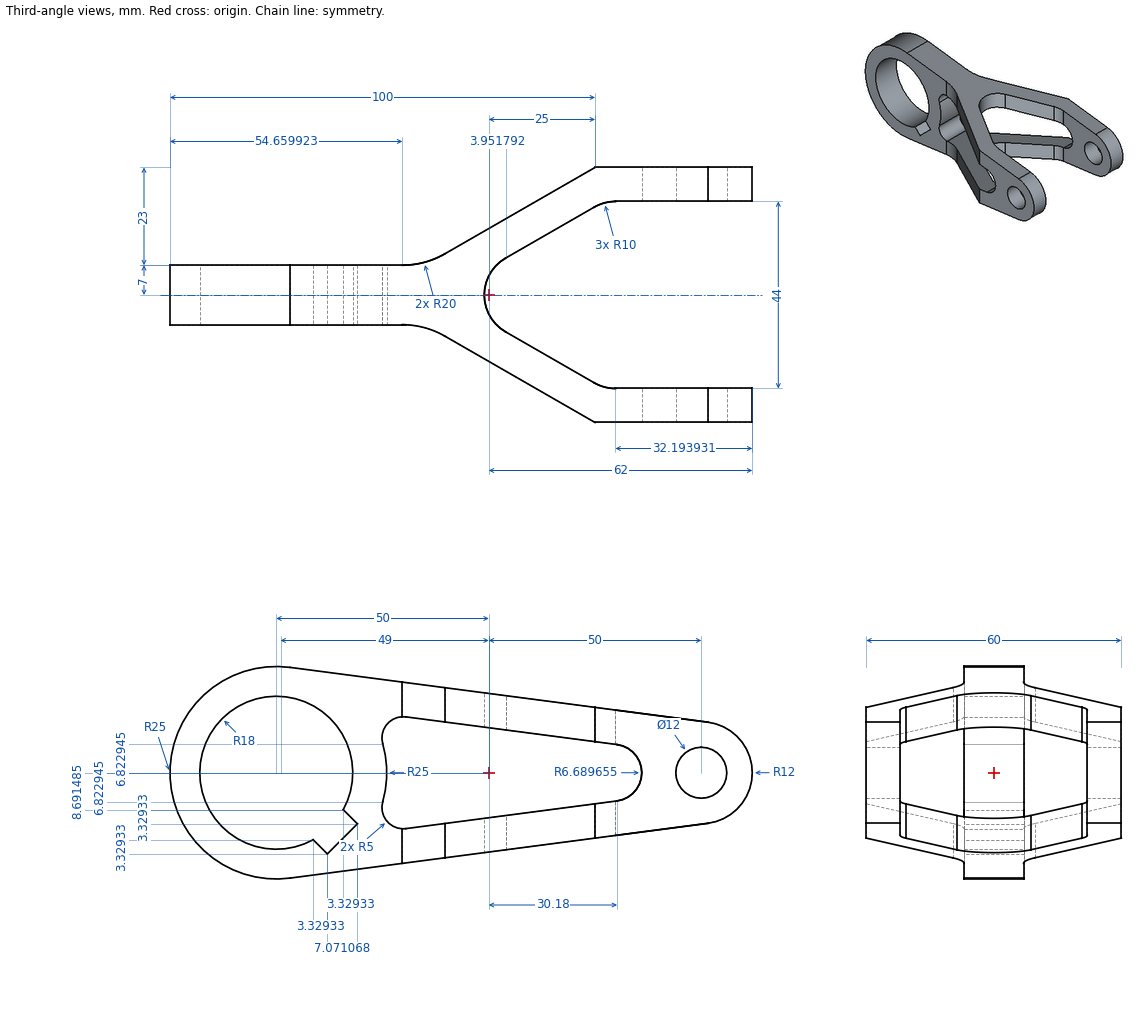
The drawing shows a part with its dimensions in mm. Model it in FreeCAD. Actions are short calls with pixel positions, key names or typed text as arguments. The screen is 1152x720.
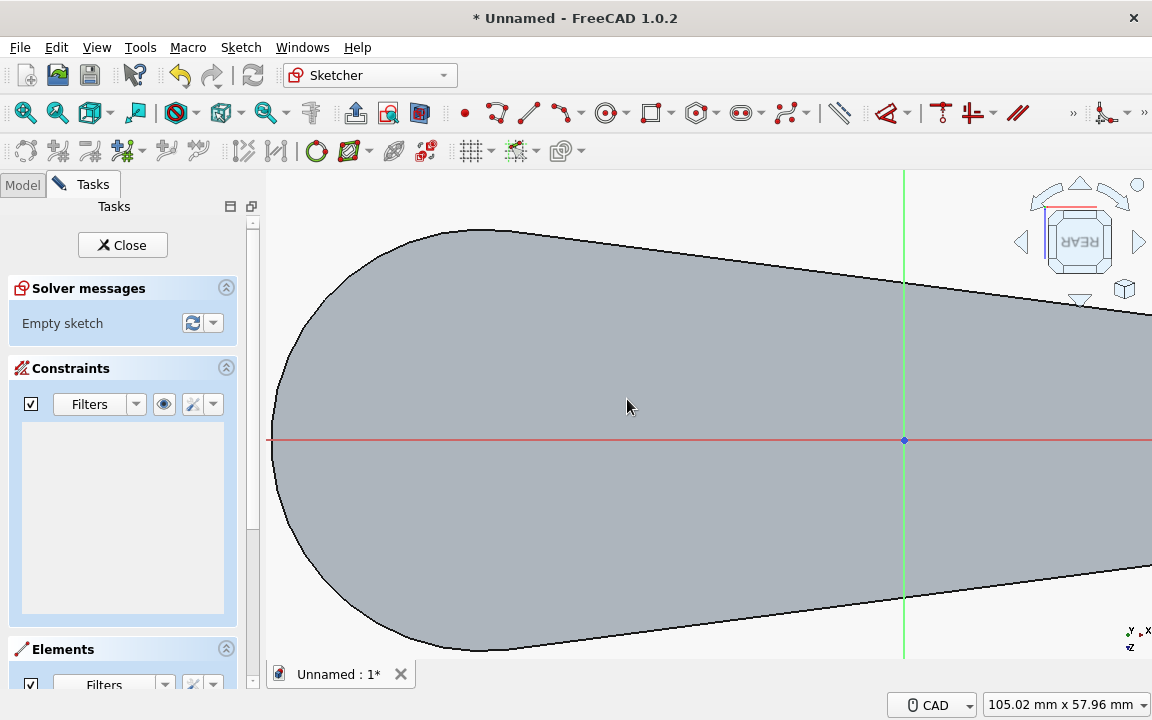
click(498, 114)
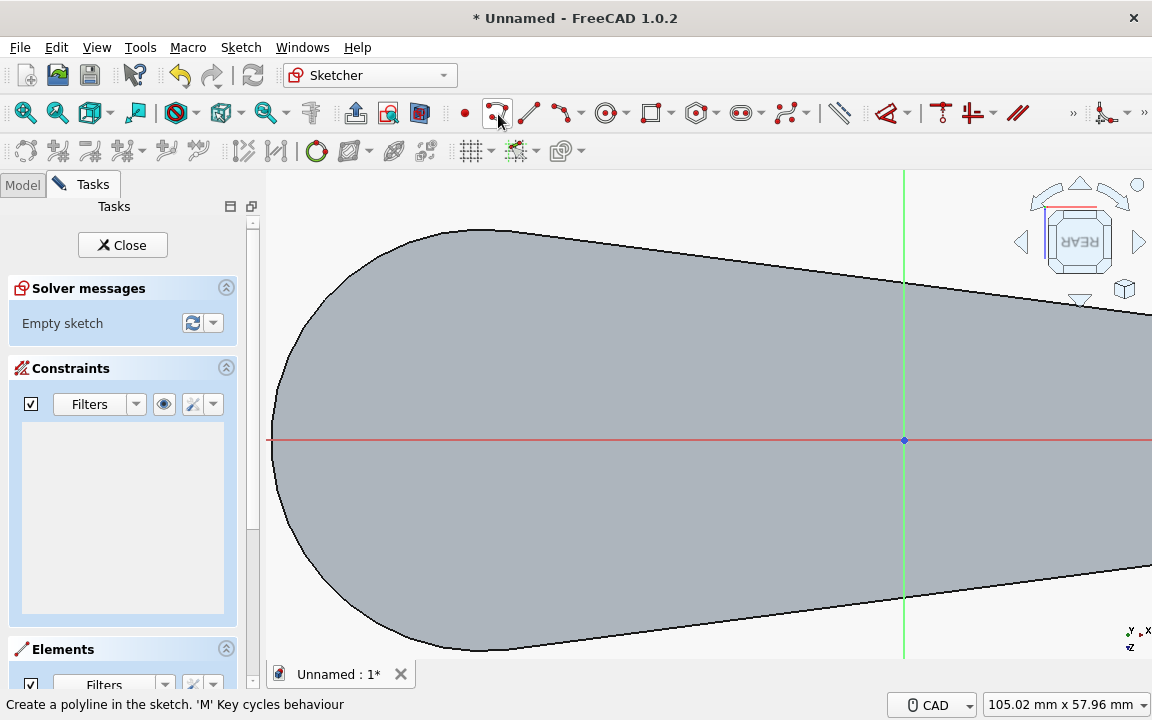
click(615, 367)
click(643, 339)
click(584, 279)
click(555, 307)
right_click(555, 307)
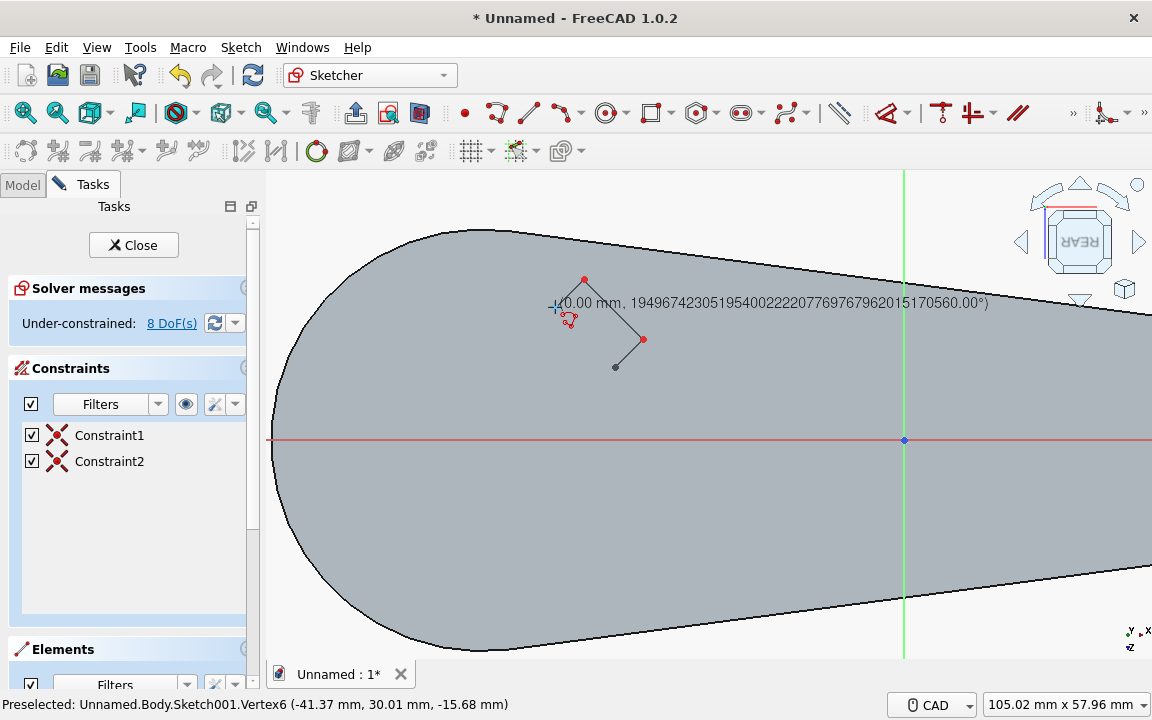
click(562, 114)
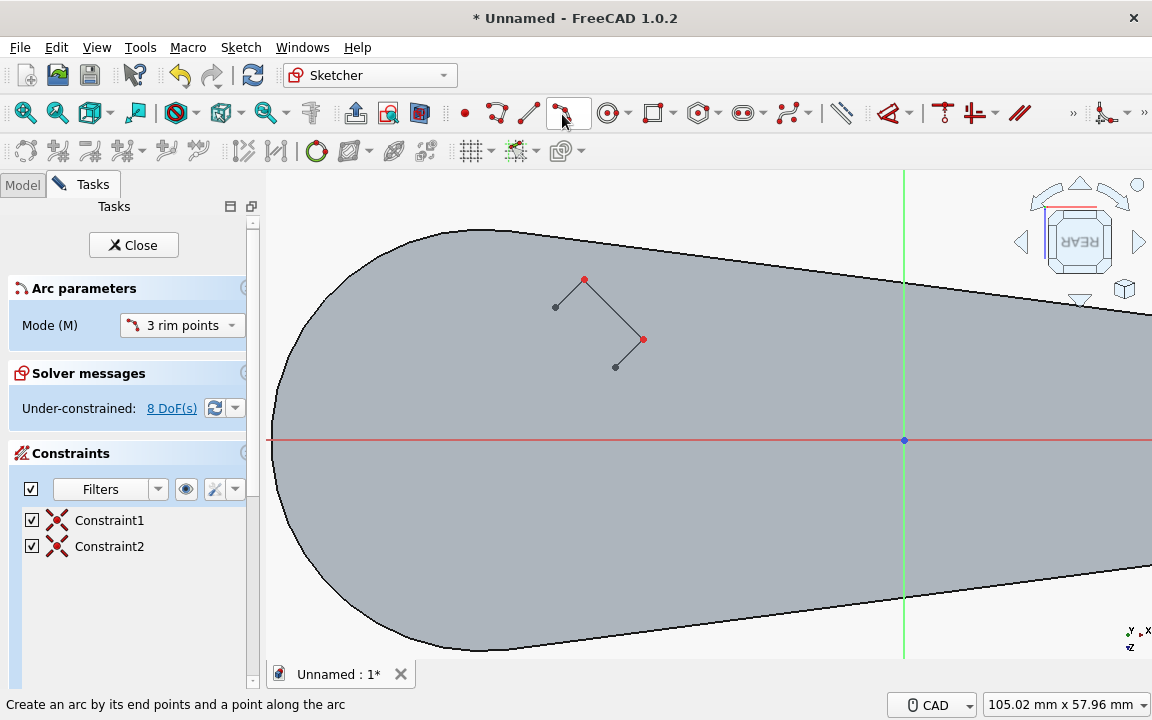
click(555, 308)
click(615, 368)
click(375, 548)
key(Escape)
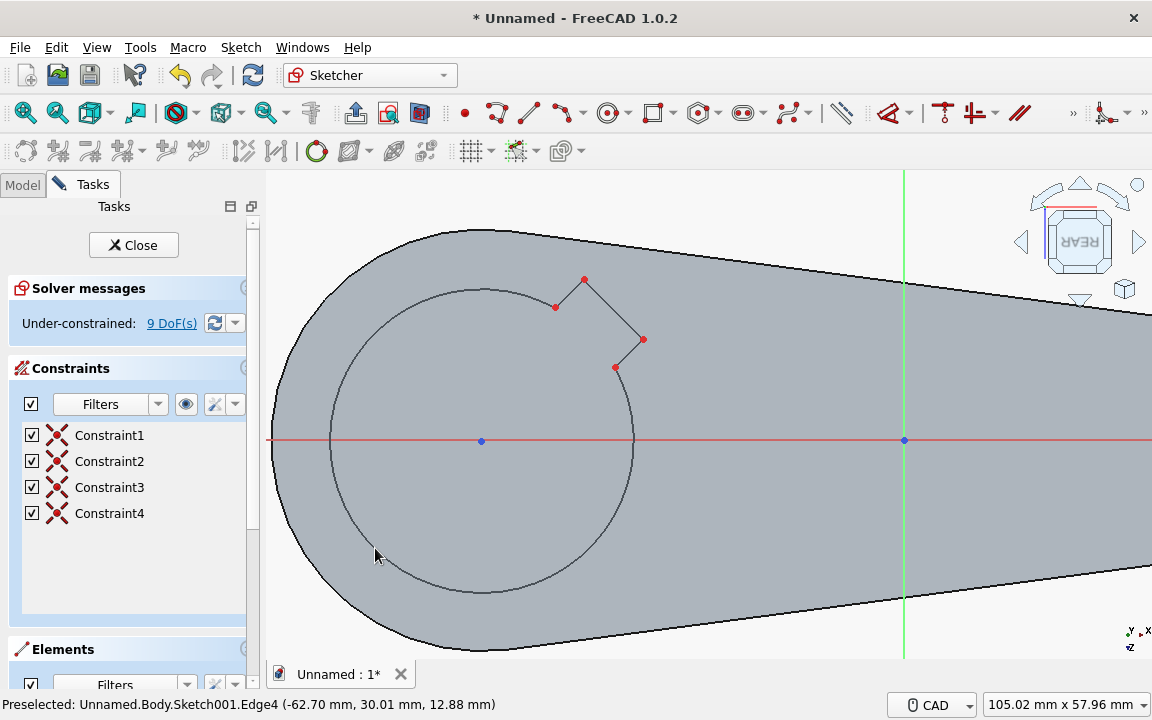
click(482, 441)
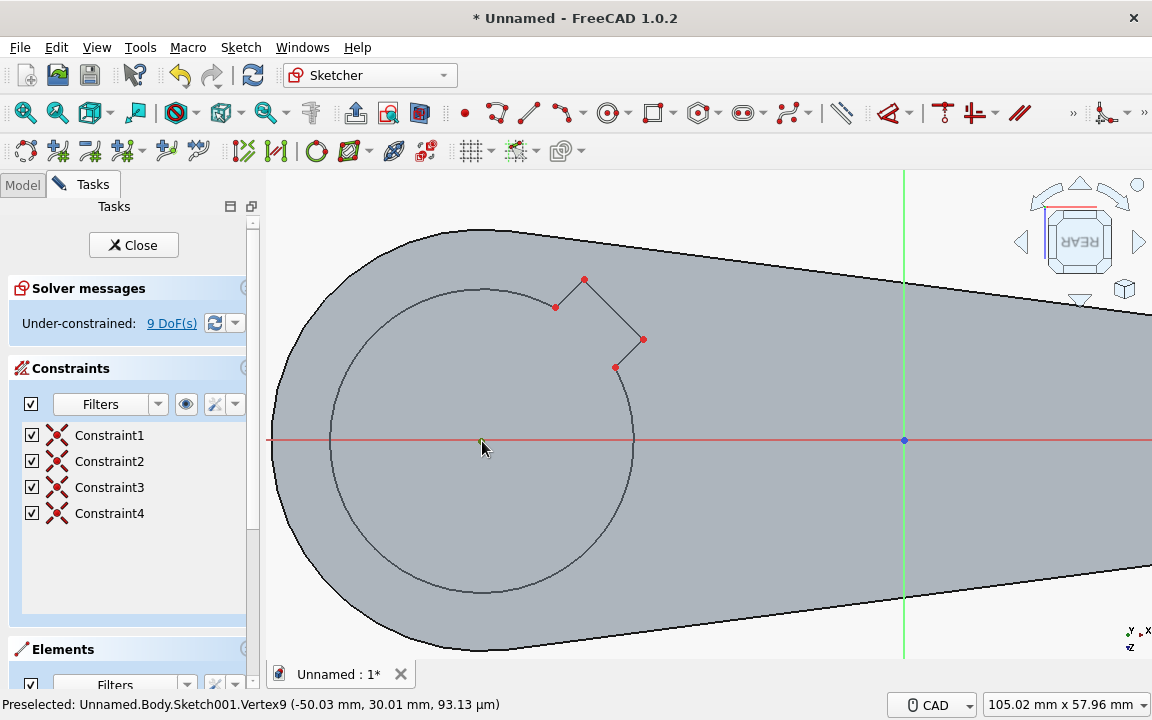
click(393, 440)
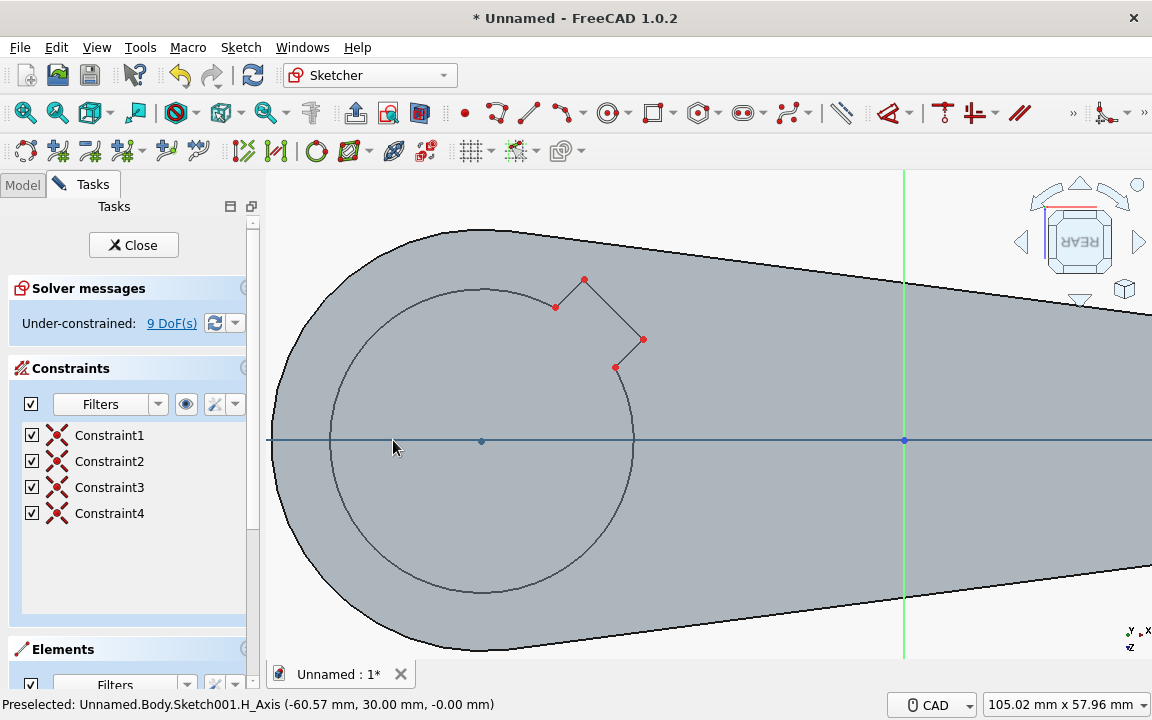
click(944, 114)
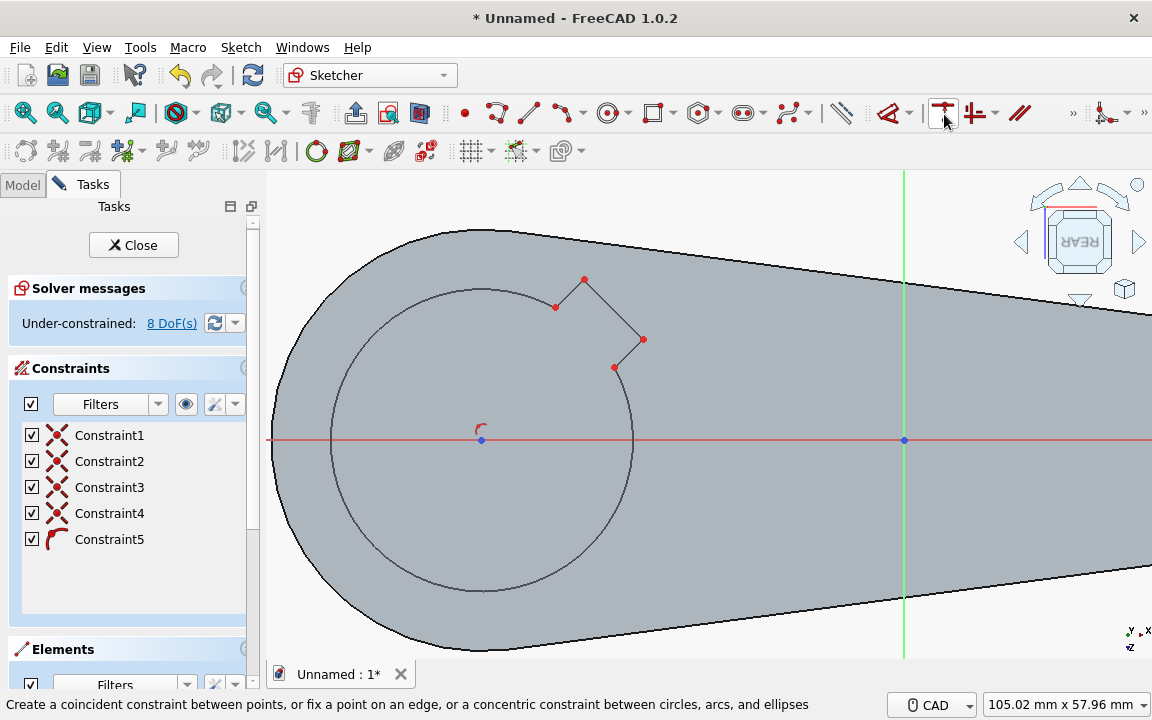
click(888, 114)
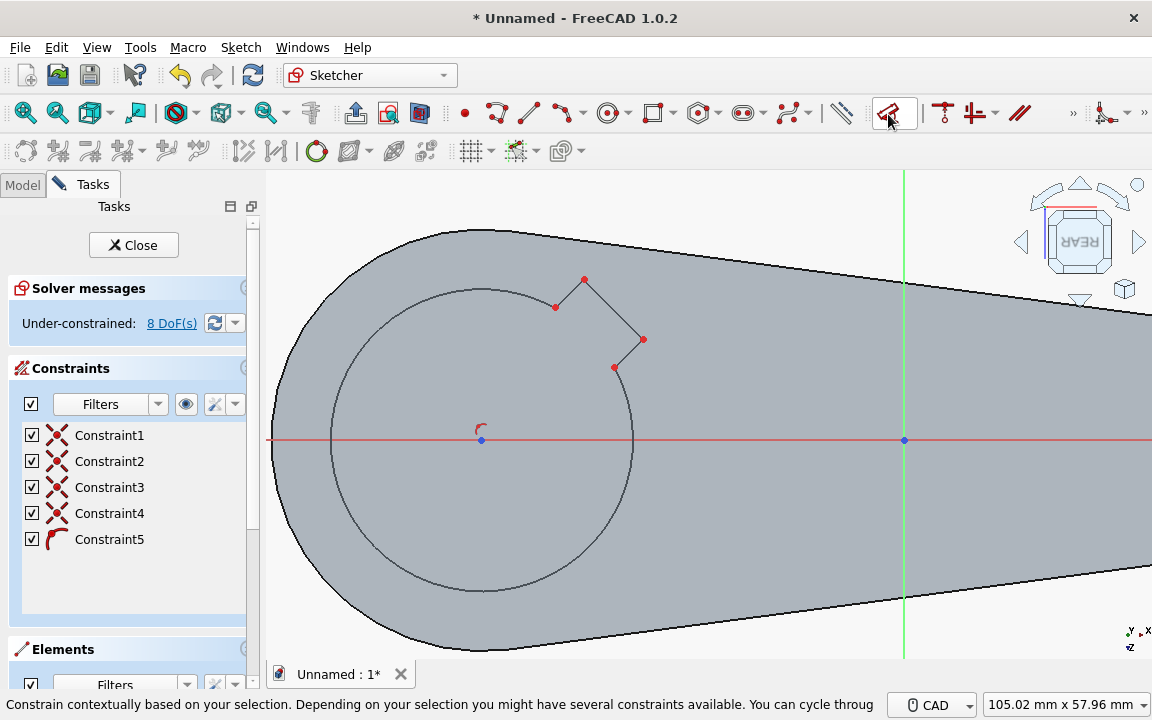
click(340, 387)
click(310, 376)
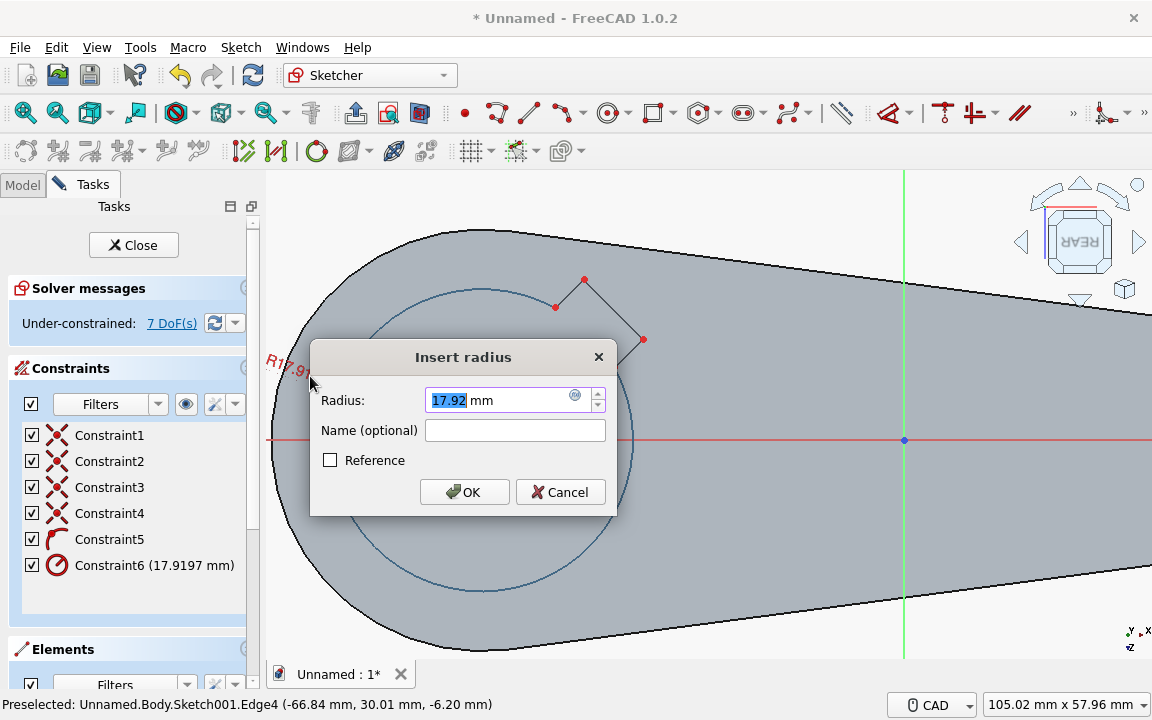
text(18)
key(Return)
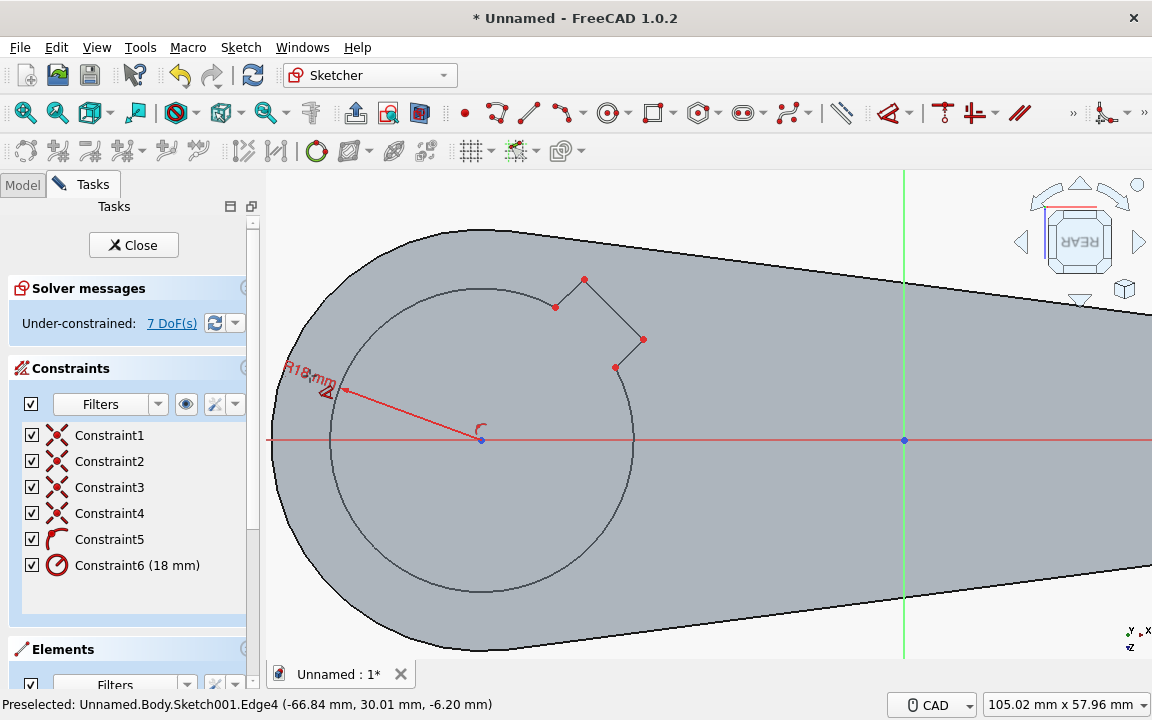
click(482, 440)
click(693, 474)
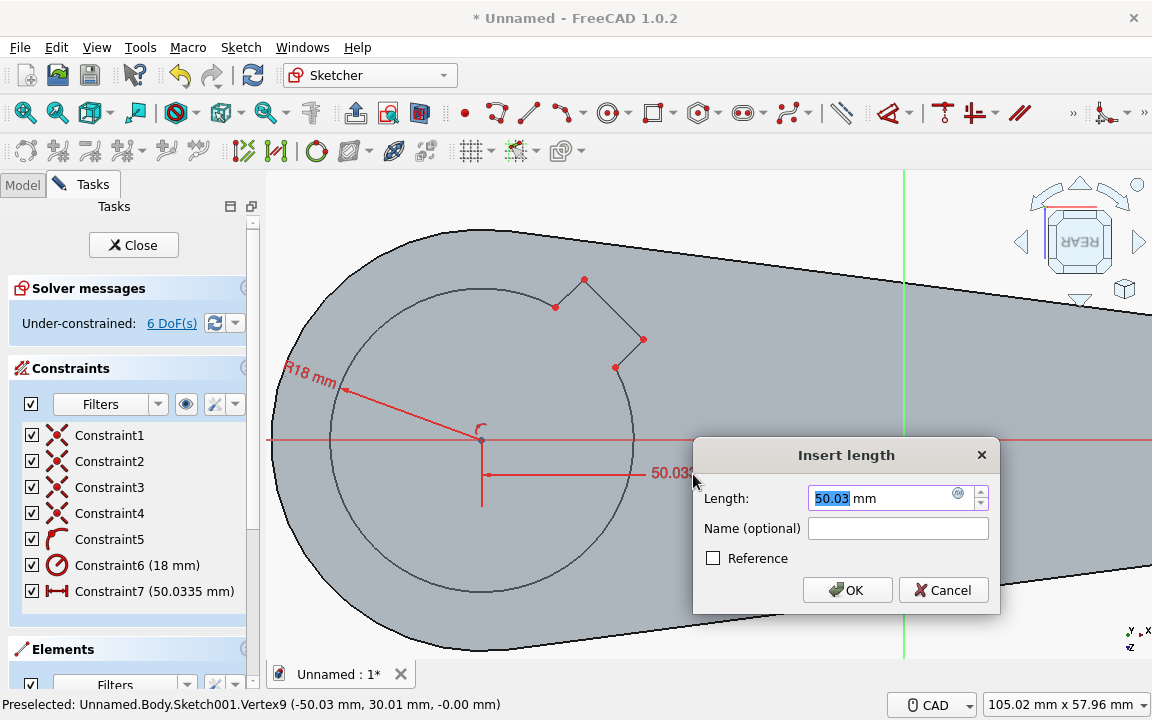
text(50)
key(Return)